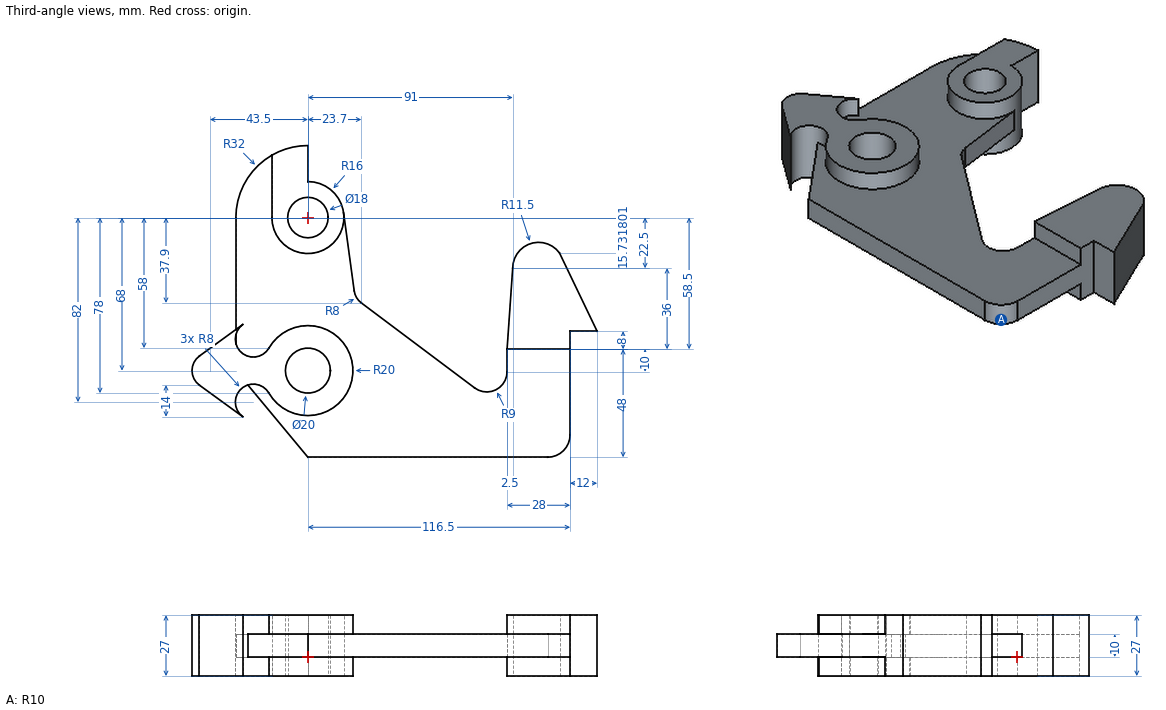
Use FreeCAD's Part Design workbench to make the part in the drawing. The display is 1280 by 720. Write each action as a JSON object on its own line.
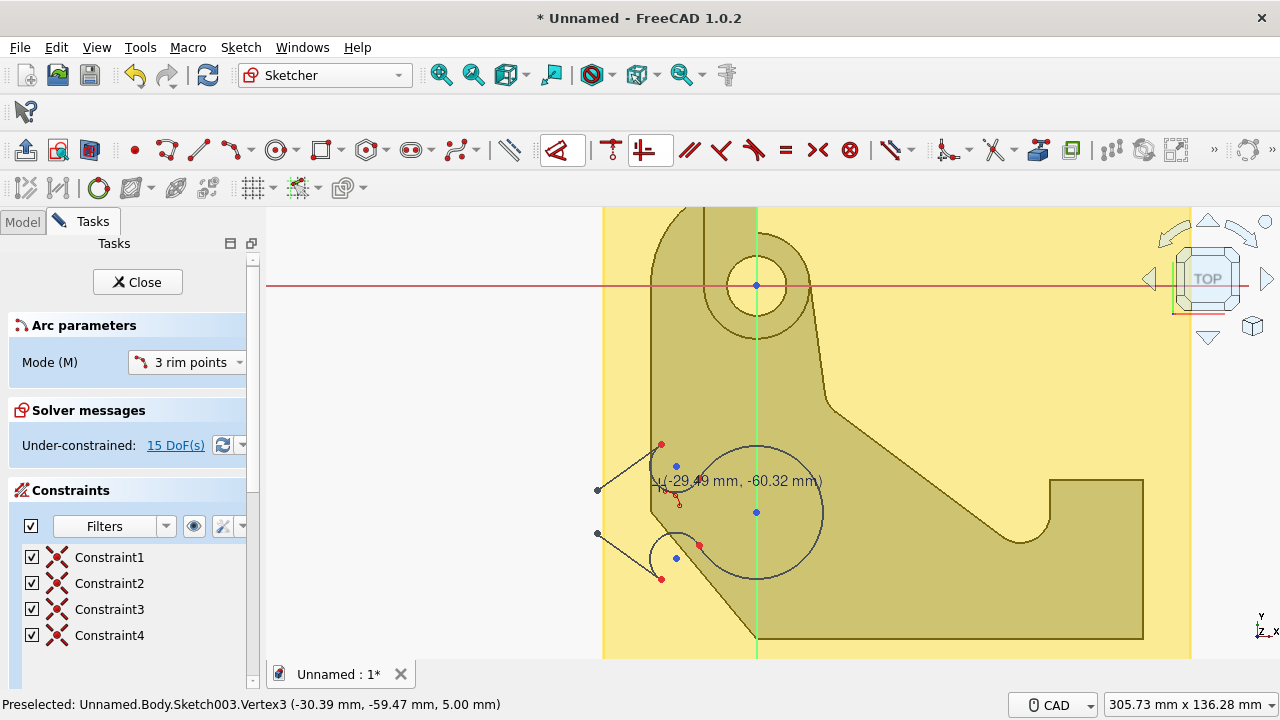
{"action": "left_click", "coordinate": [597, 491]}
{"action": "left_click", "coordinate": [597, 534]}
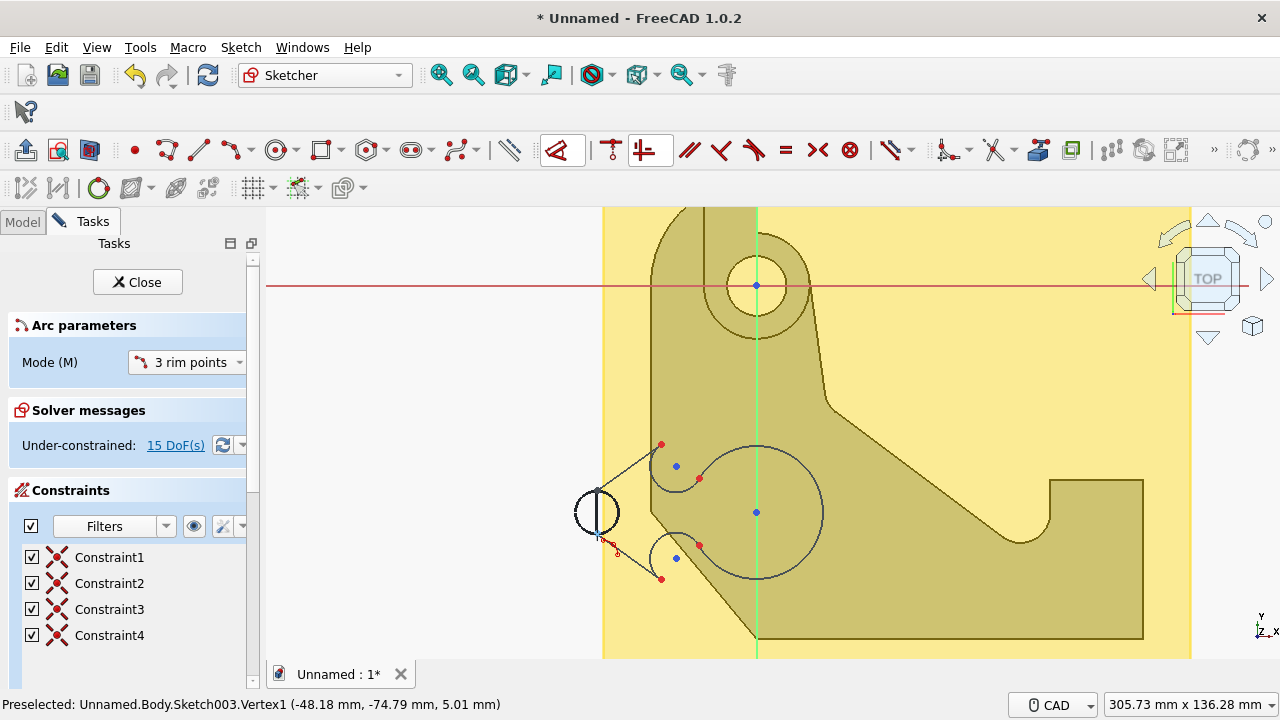
{"action": "scroll", "coordinate": [586, 511], "scroll_direction": "up", "scroll_amount": 2}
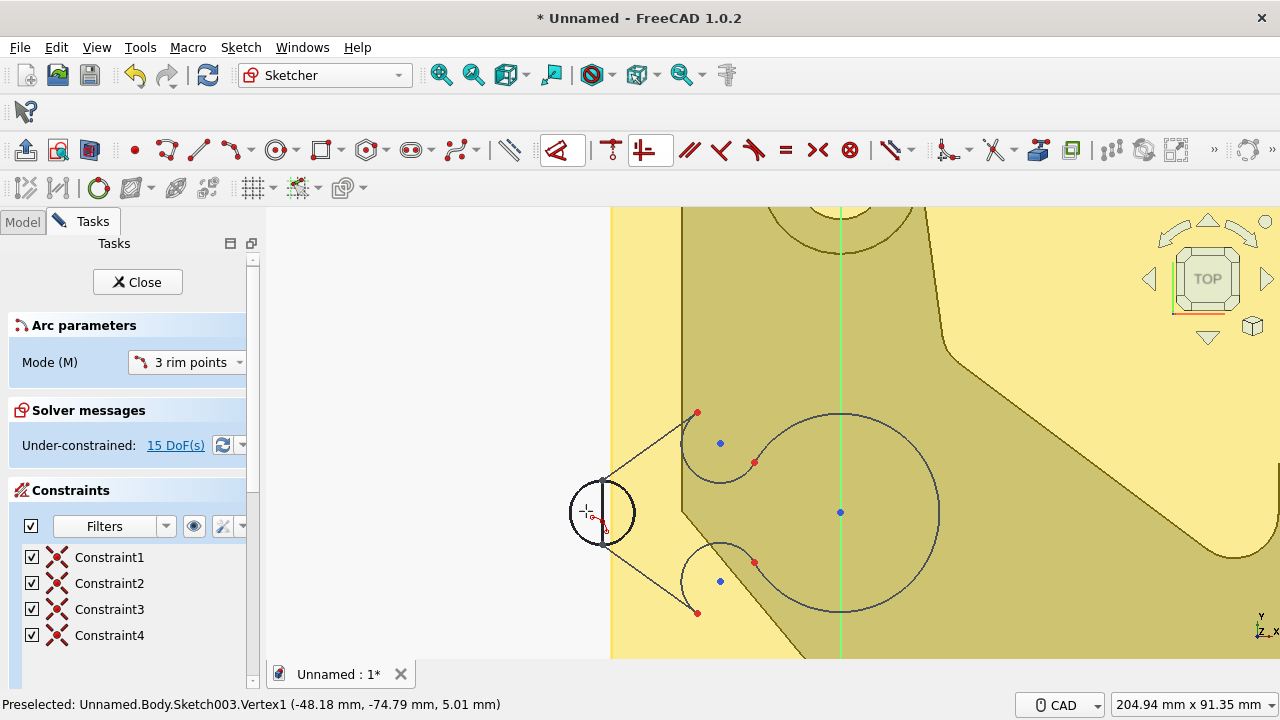
{"action": "left_click", "coordinate": [586, 511]}
{"action": "key", "text": "Escape"}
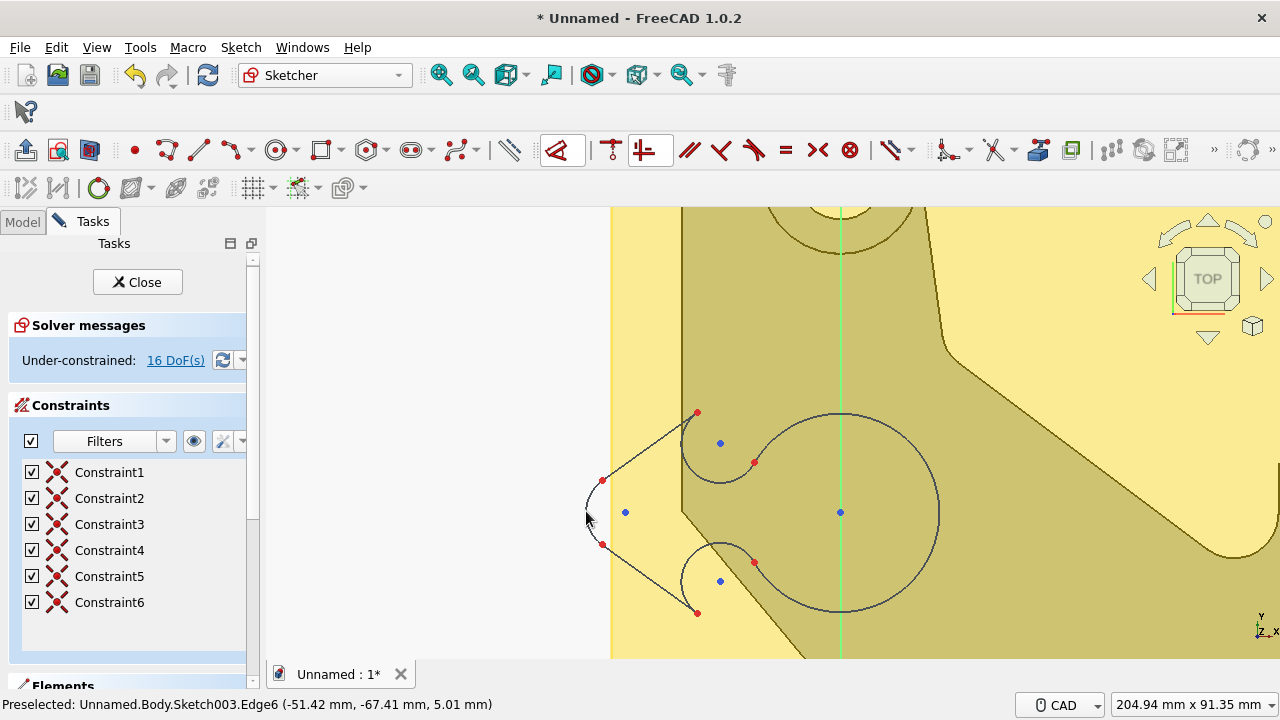
{"action": "left_click", "coordinate": [631, 566]}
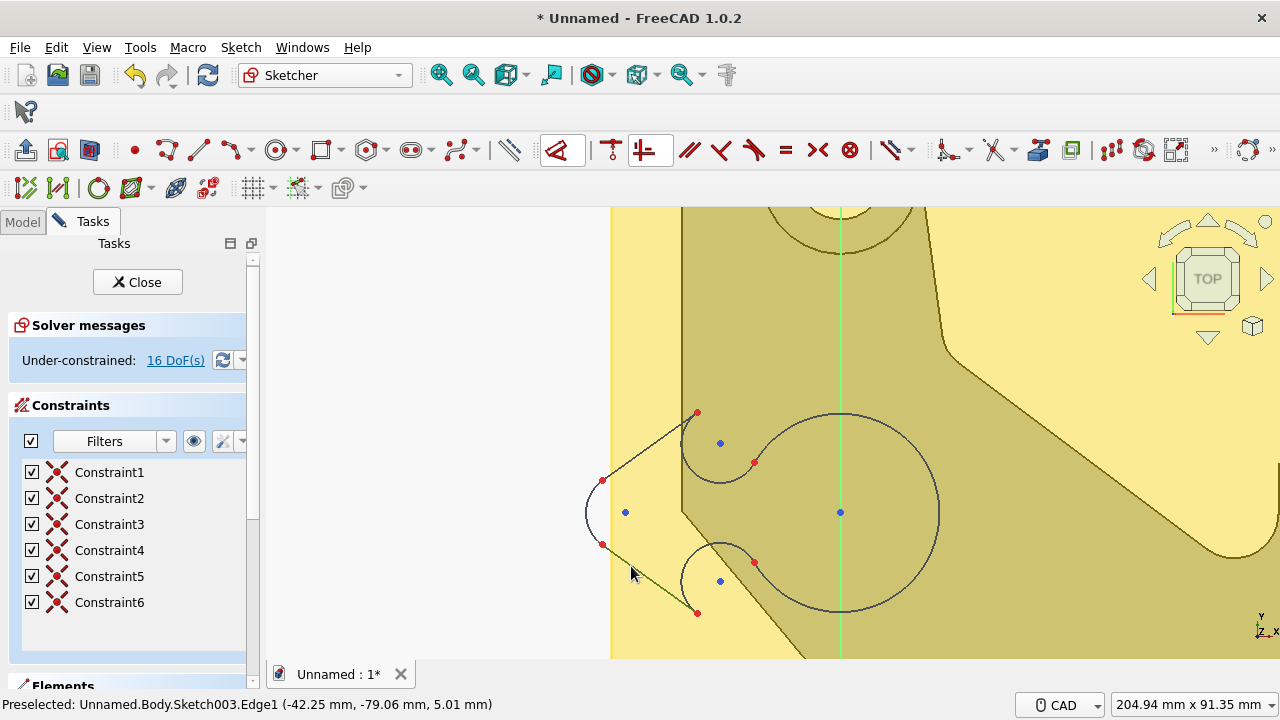
{"action": "left_click", "coordinate": [720, 543]}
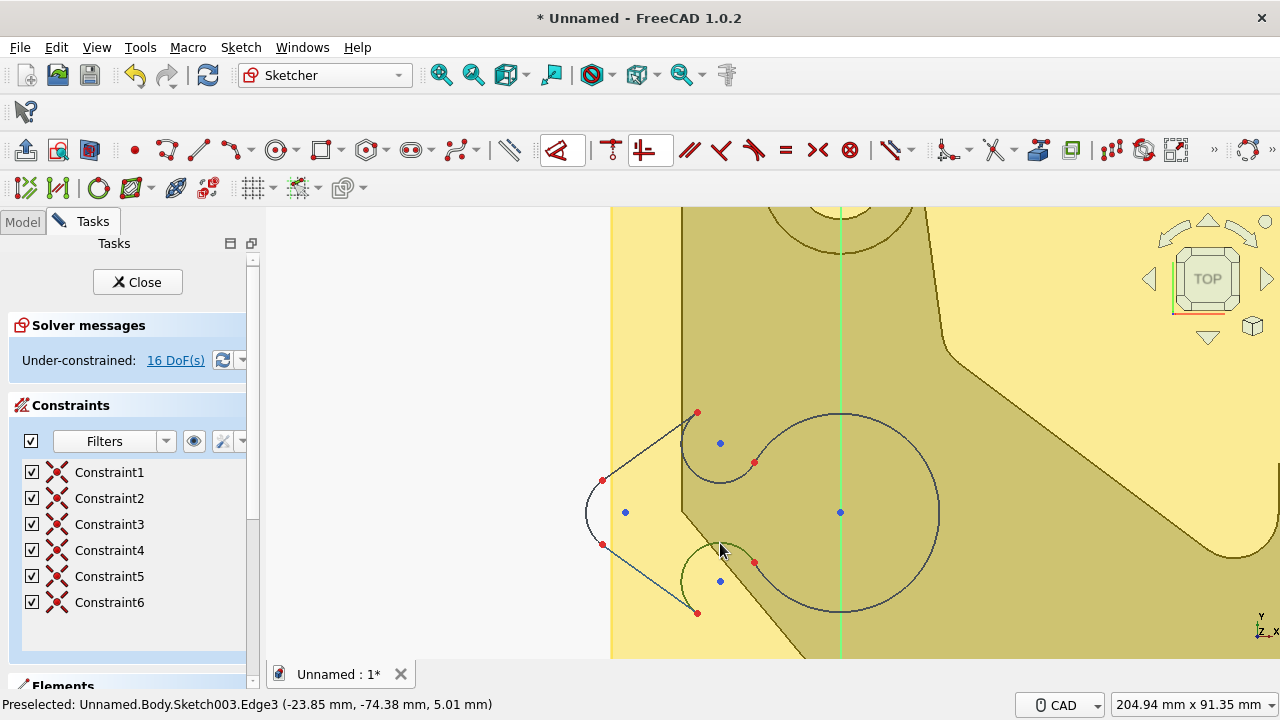
{"action": "left_click", "coordinate": [754, 150]}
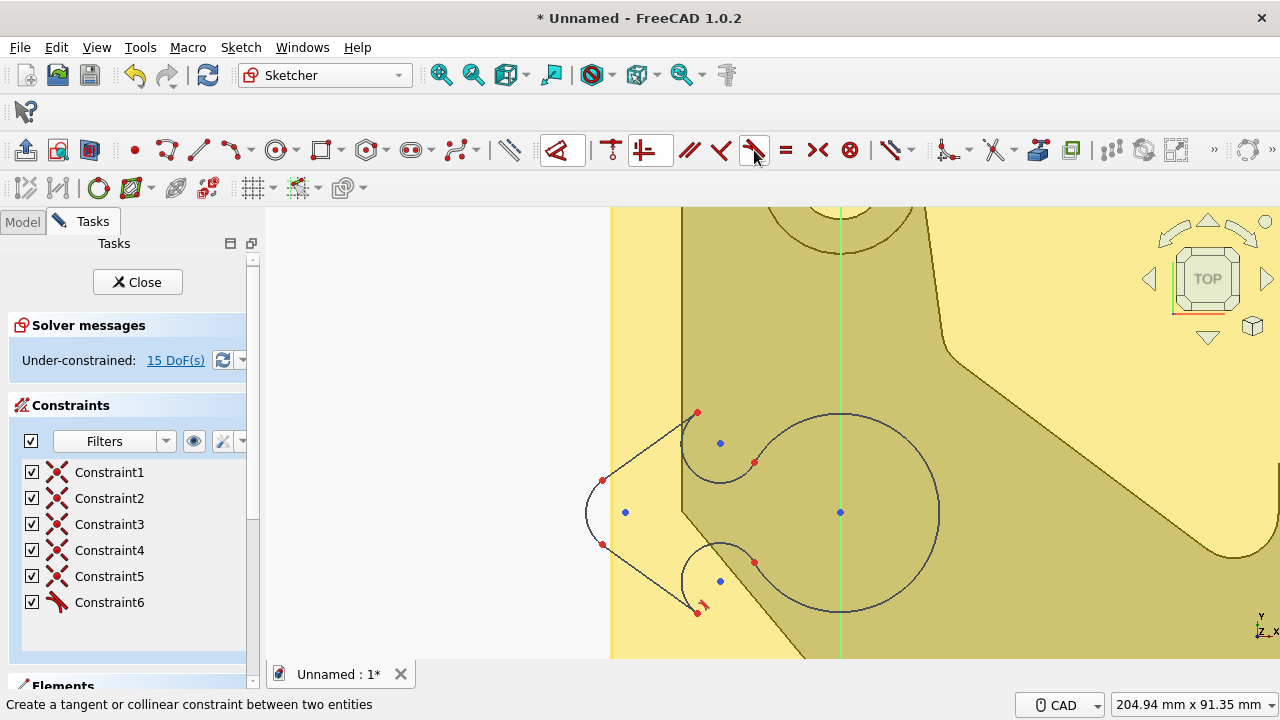
{"action": "left_click", "coordinate": [631, 566]}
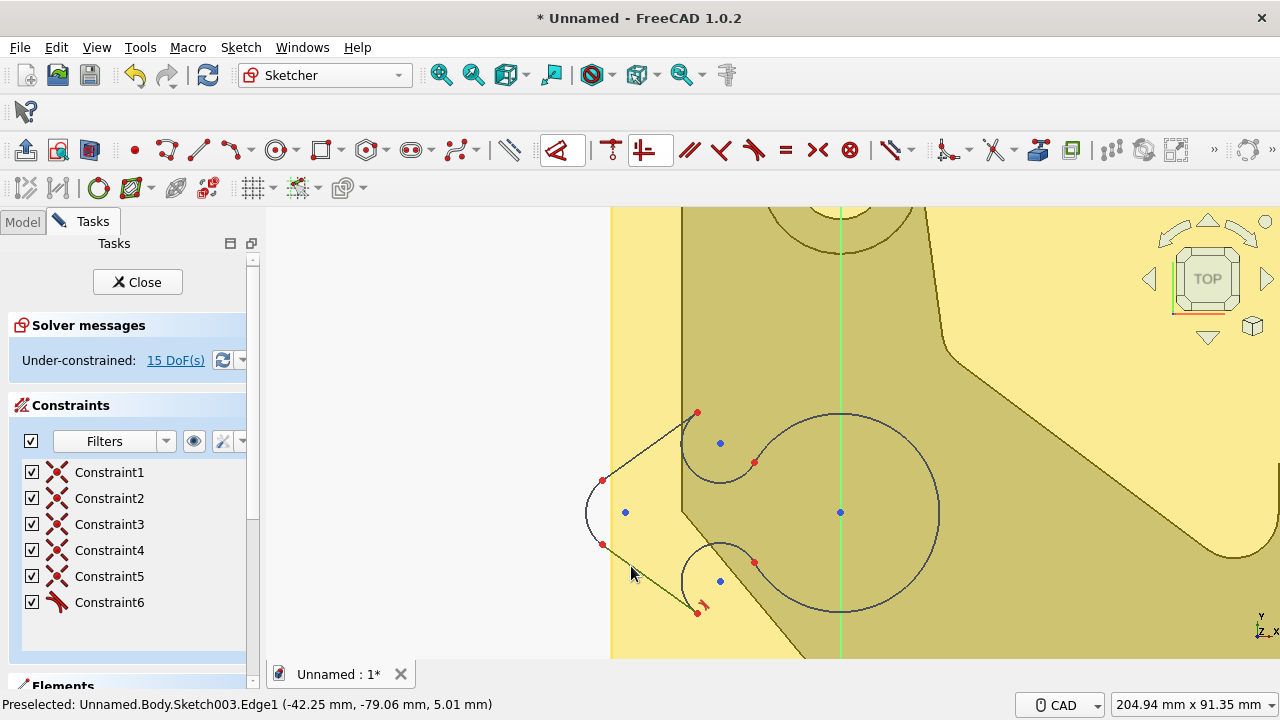
{"action": "left_click", "coordinate": [589, 498]}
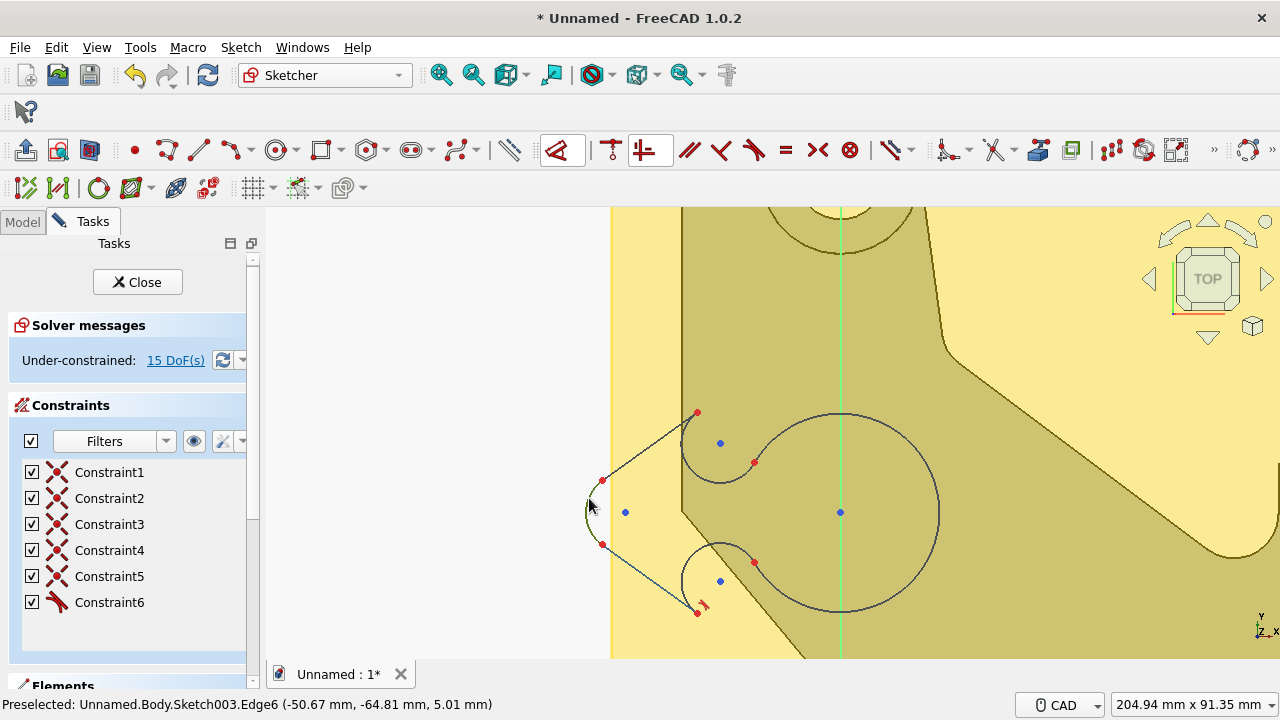
{"action": "left_click", "coordinate": [754, 150]}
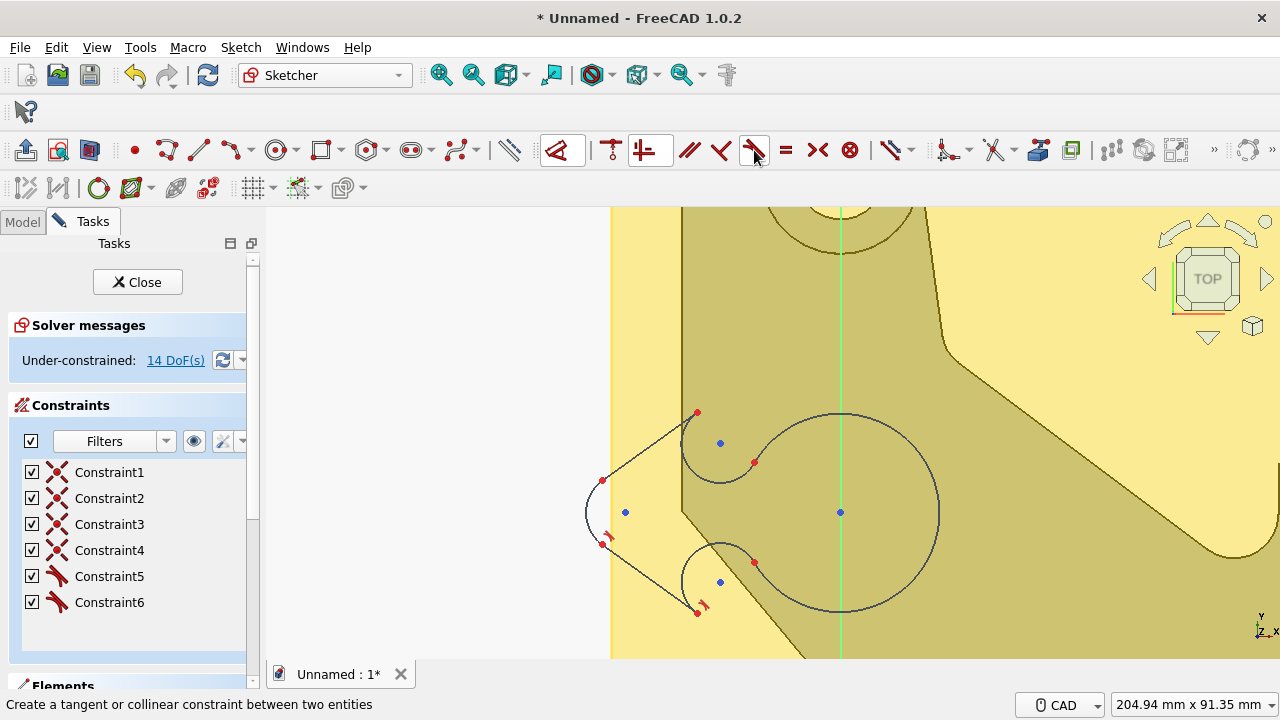
{"action": "left_click", "coordinate": [669, 433]}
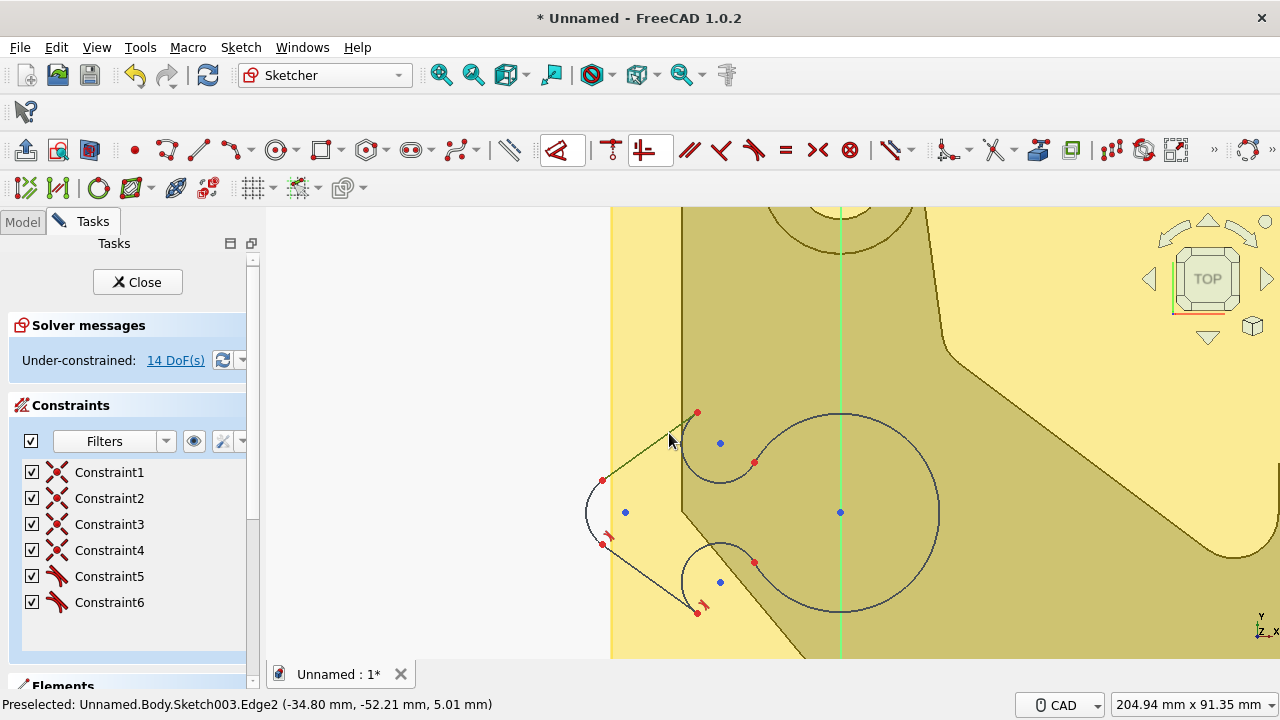
{"action": "left_click", "coordinate": [682, 449]}